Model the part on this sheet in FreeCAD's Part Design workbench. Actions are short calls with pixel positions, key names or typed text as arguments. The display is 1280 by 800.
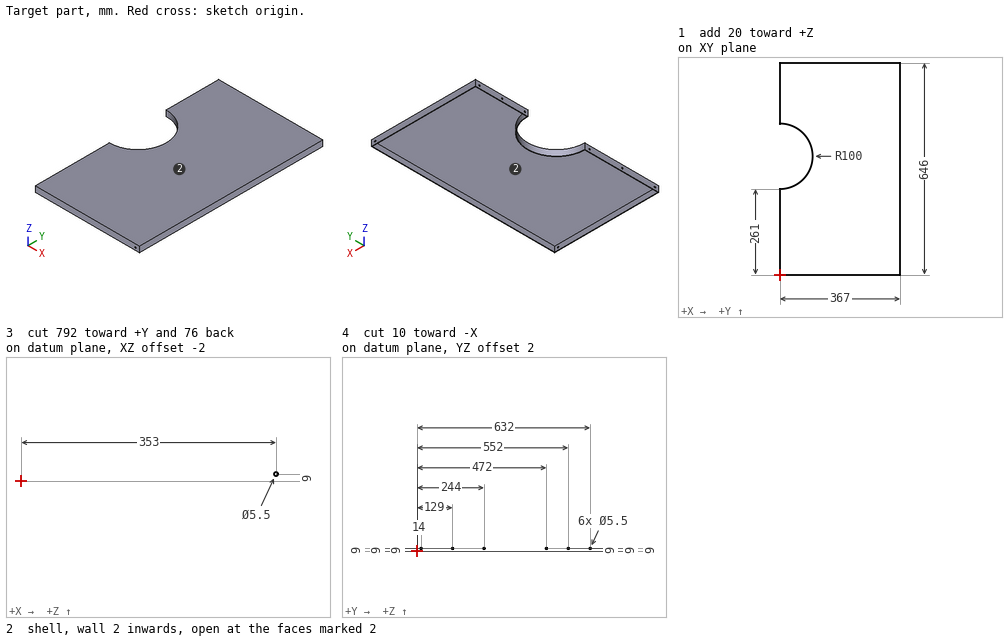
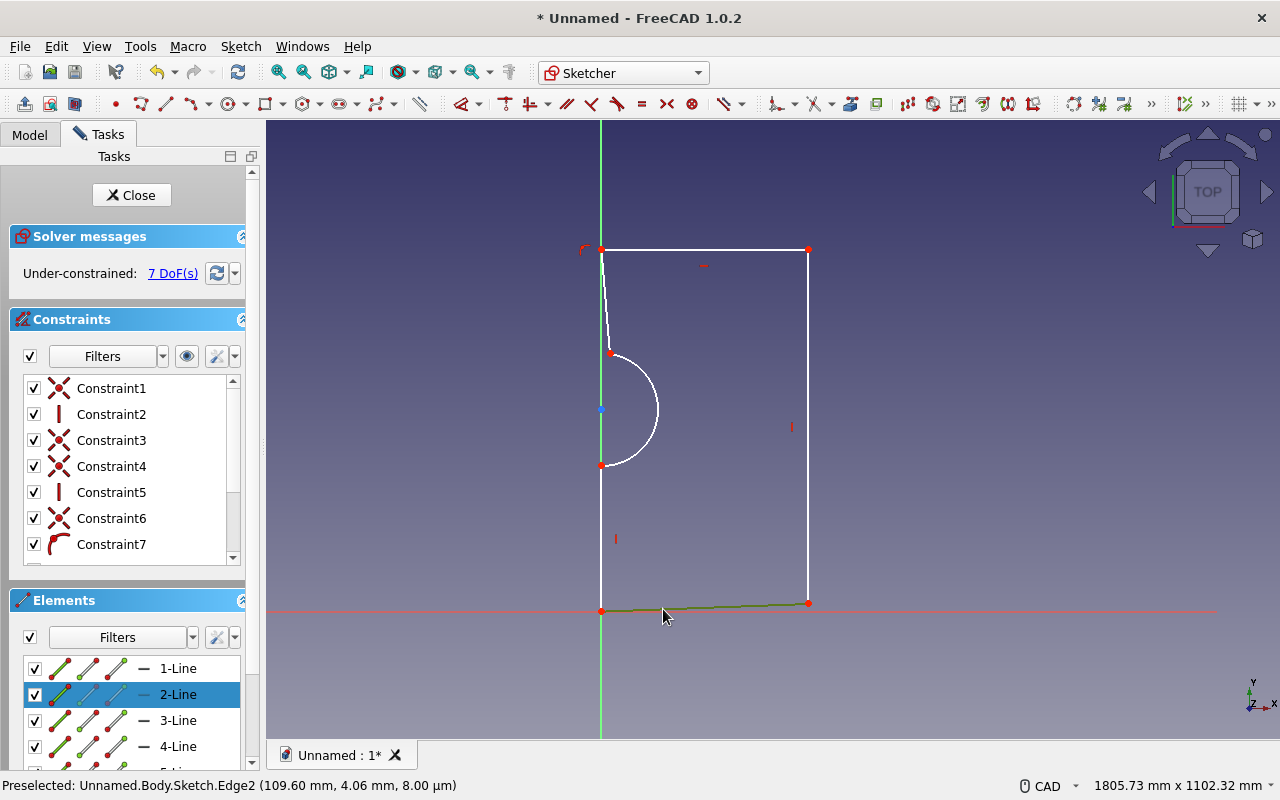
key(h)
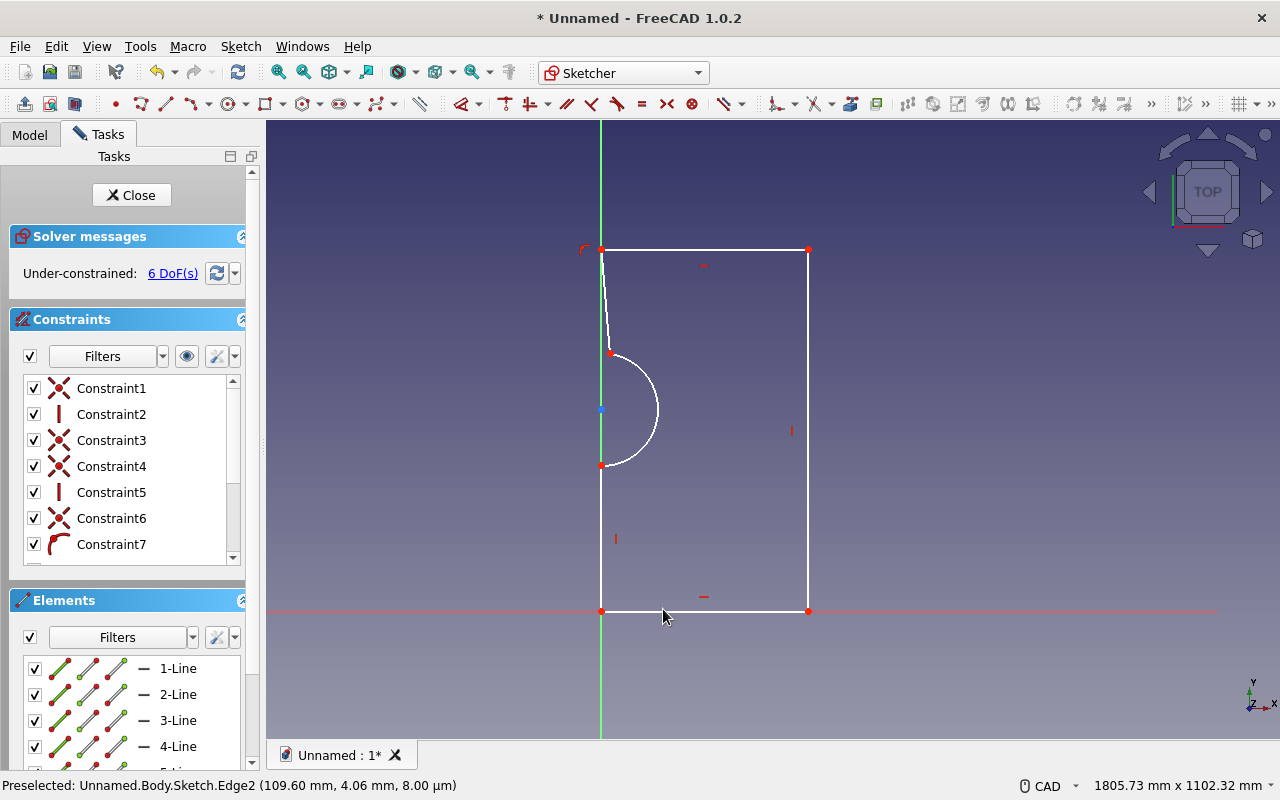
click(604, 281)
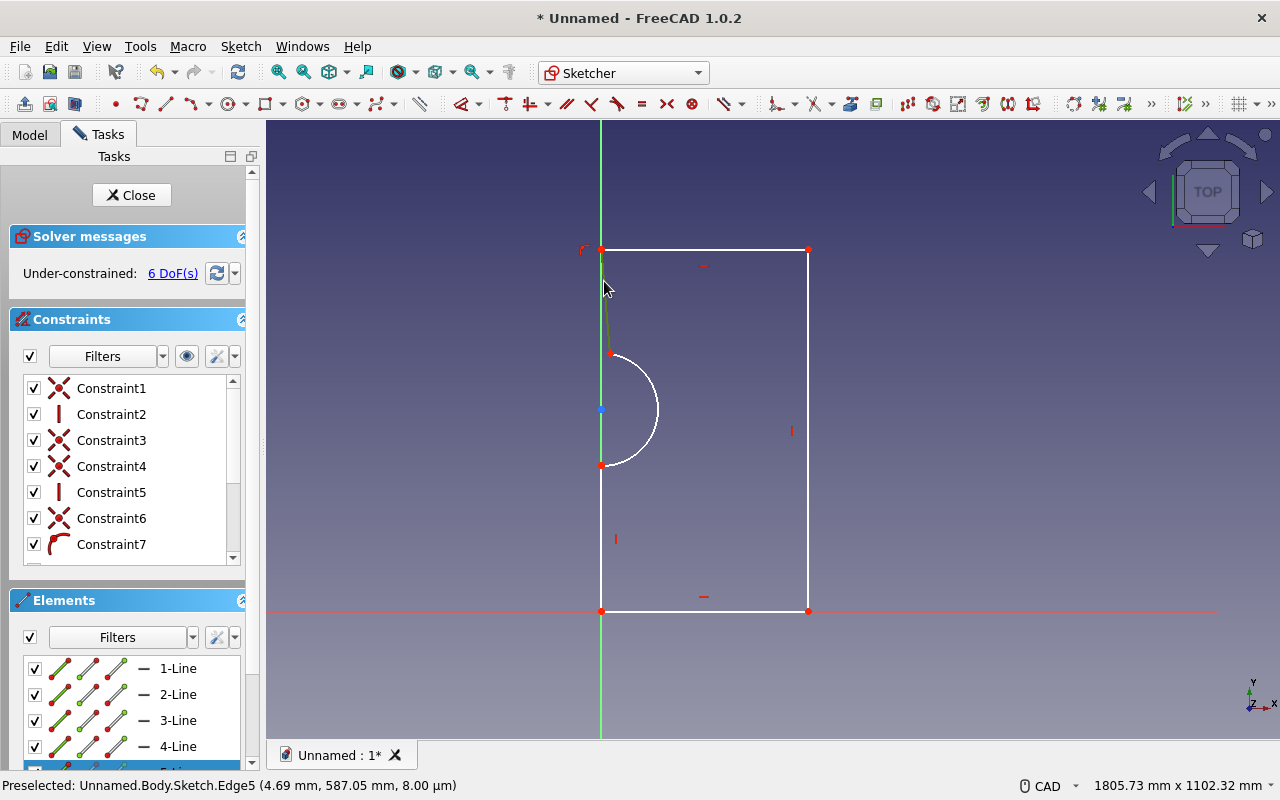
key(v)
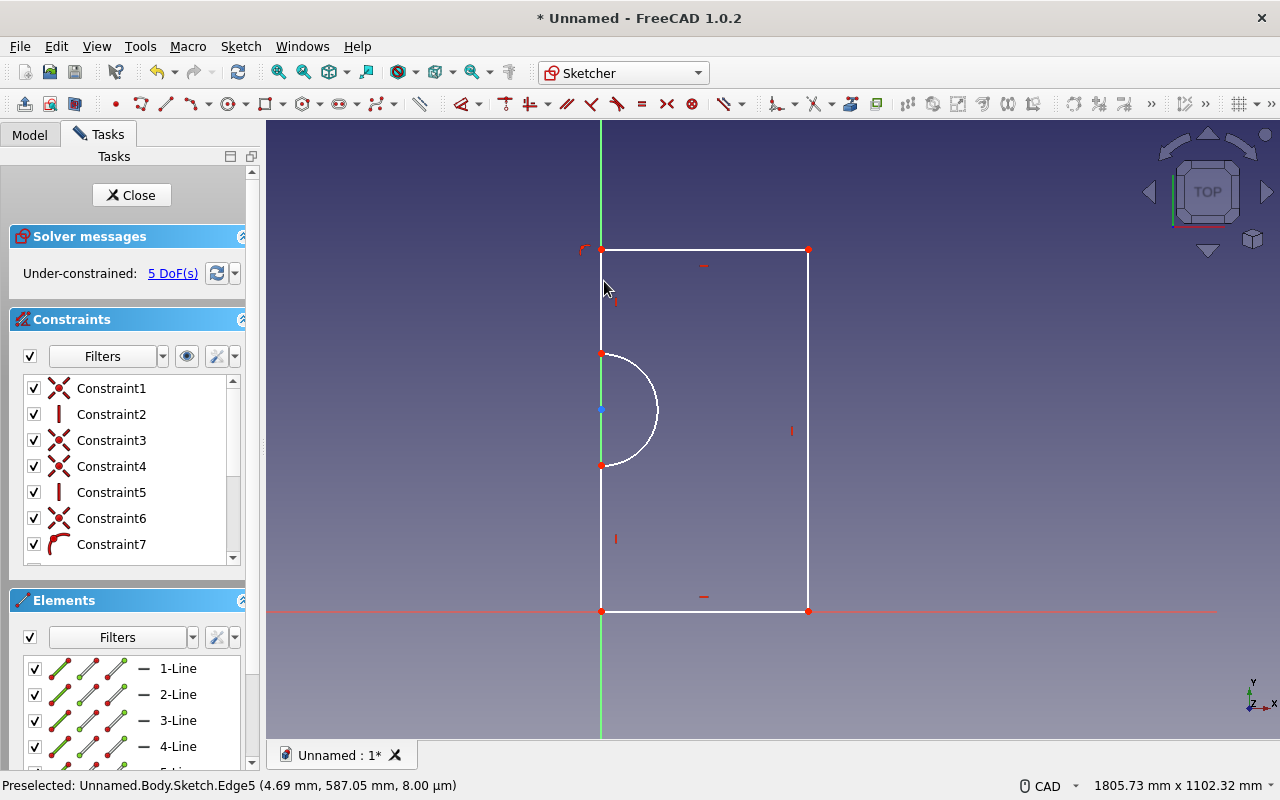
click(602, 410)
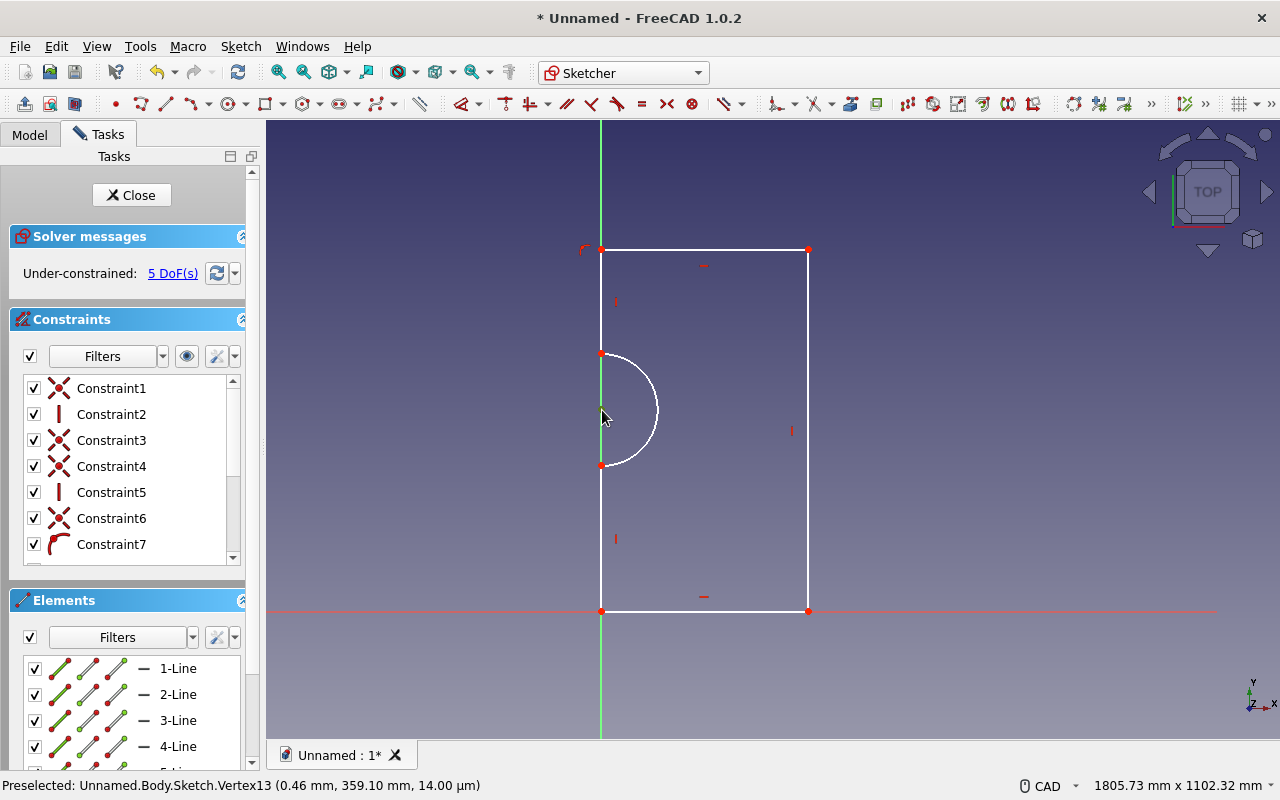
click(601, 671)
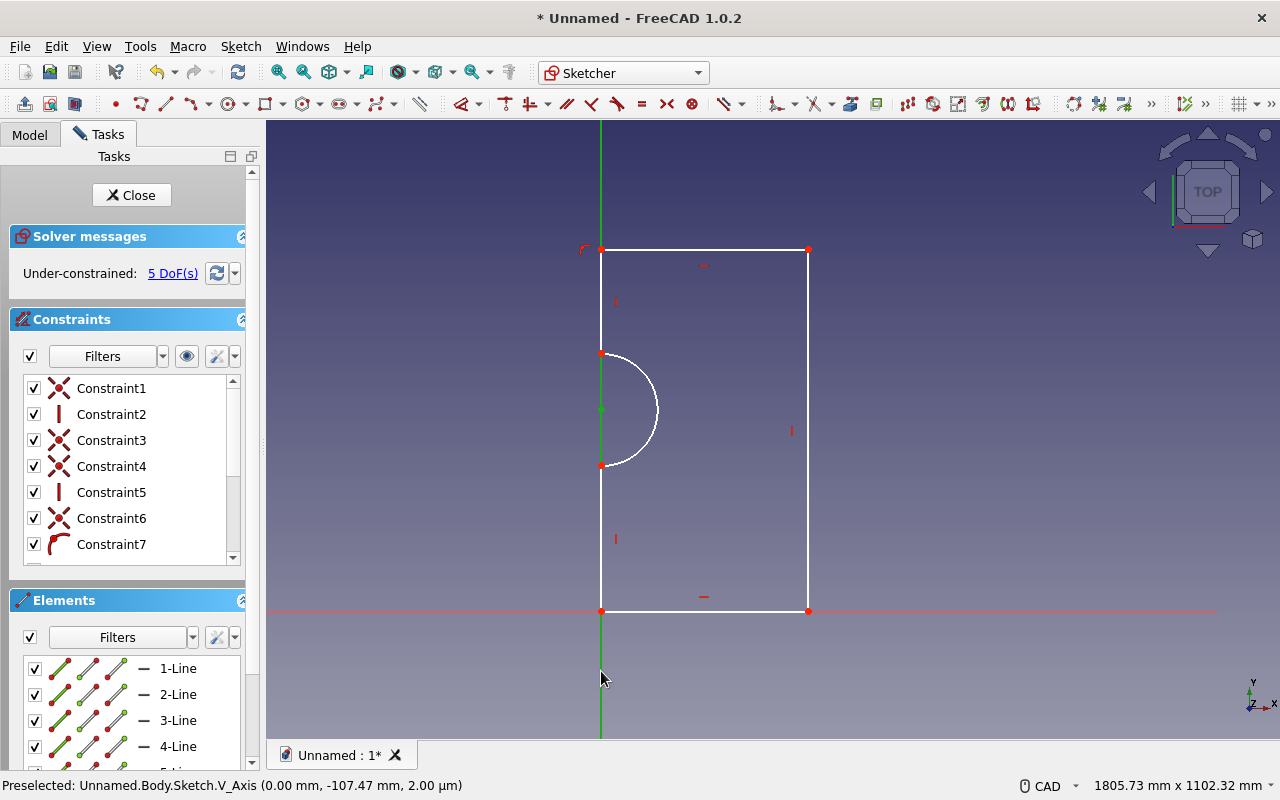
click(505, 104)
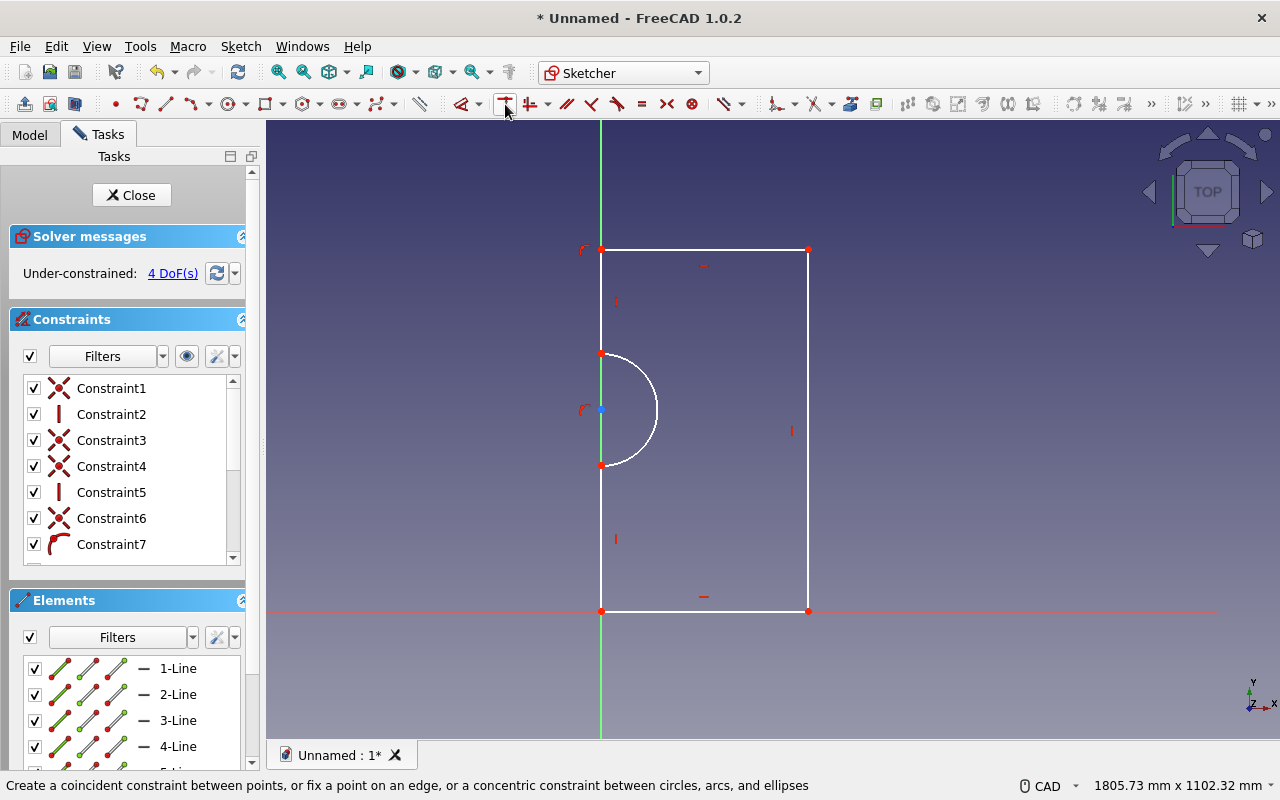
click(460, 104)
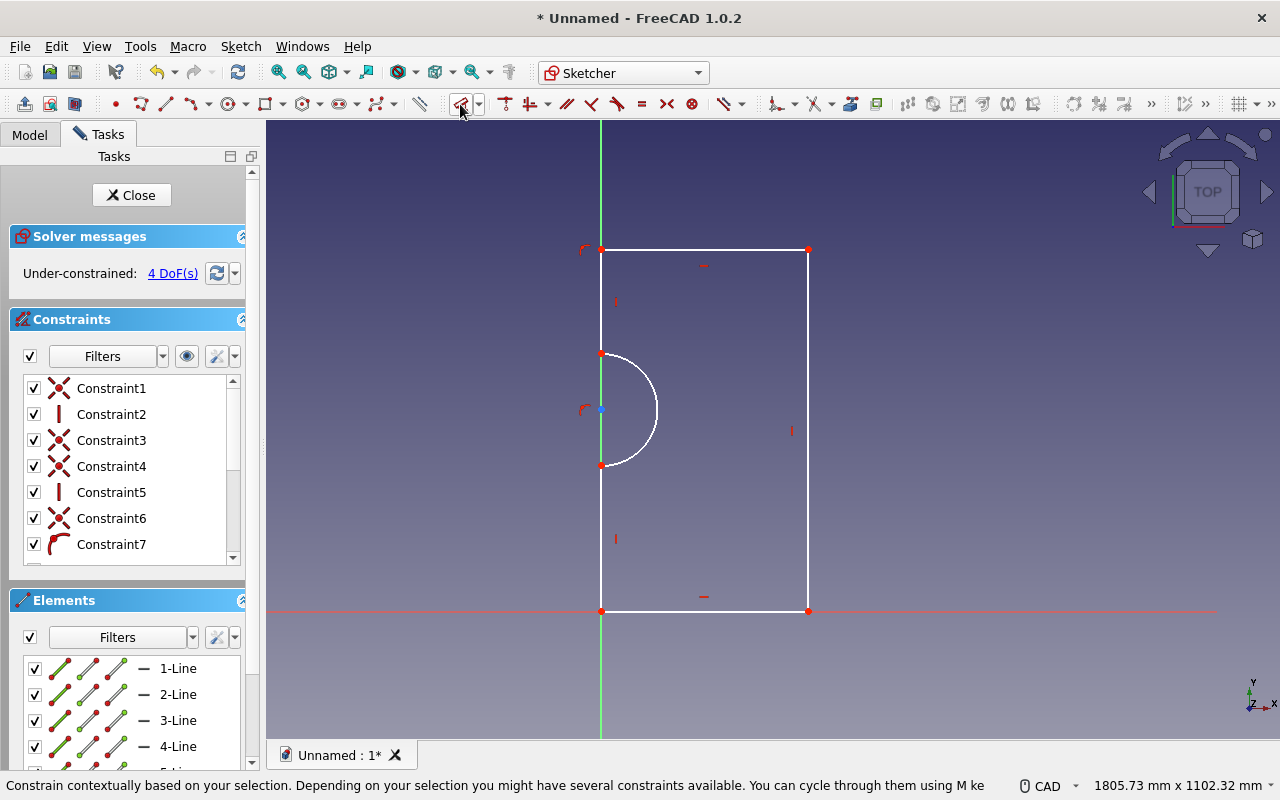
click(647, 443)
click(673, 462)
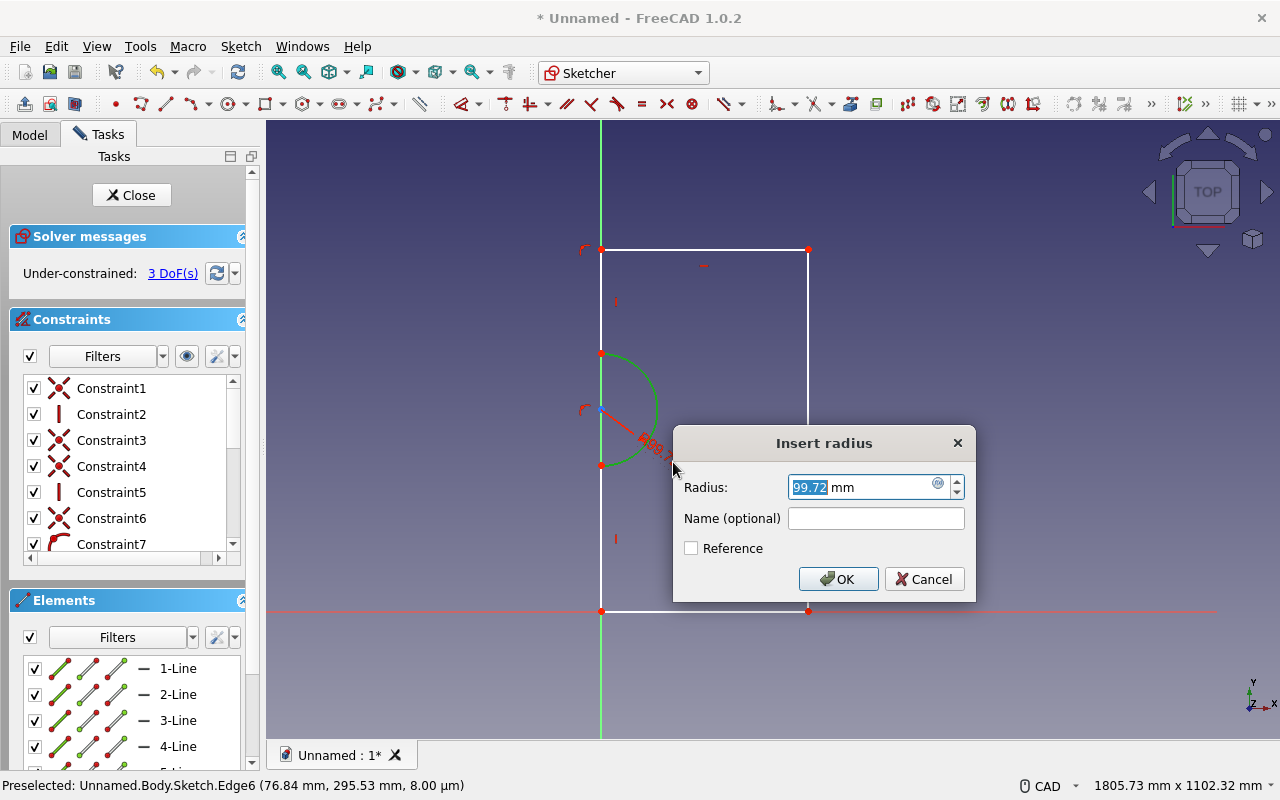
text(100)
key(Return)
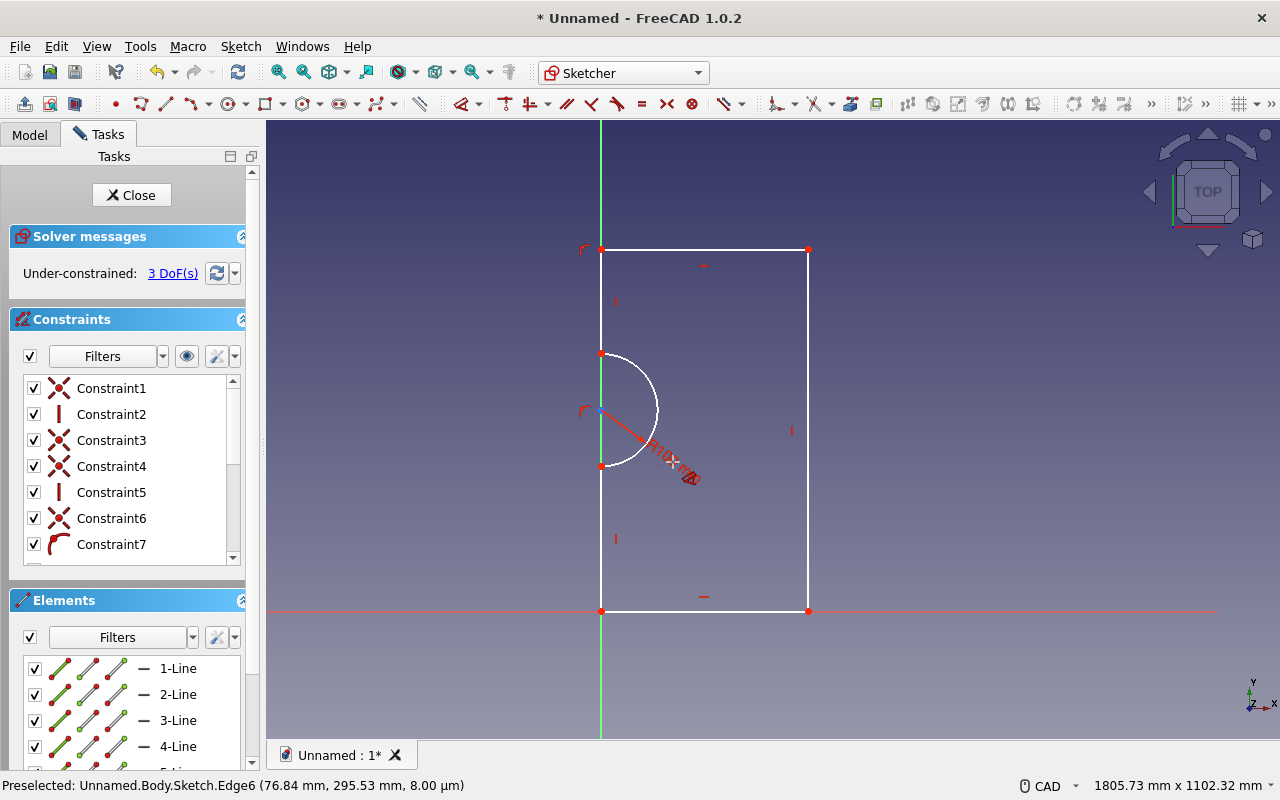
click(601, 510)
click(567, 539)